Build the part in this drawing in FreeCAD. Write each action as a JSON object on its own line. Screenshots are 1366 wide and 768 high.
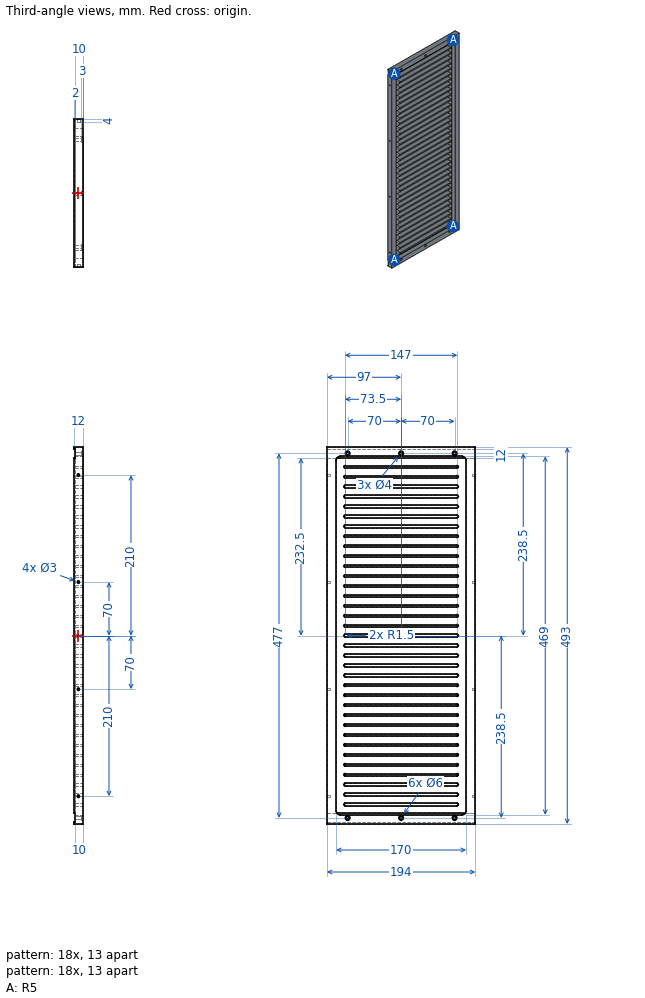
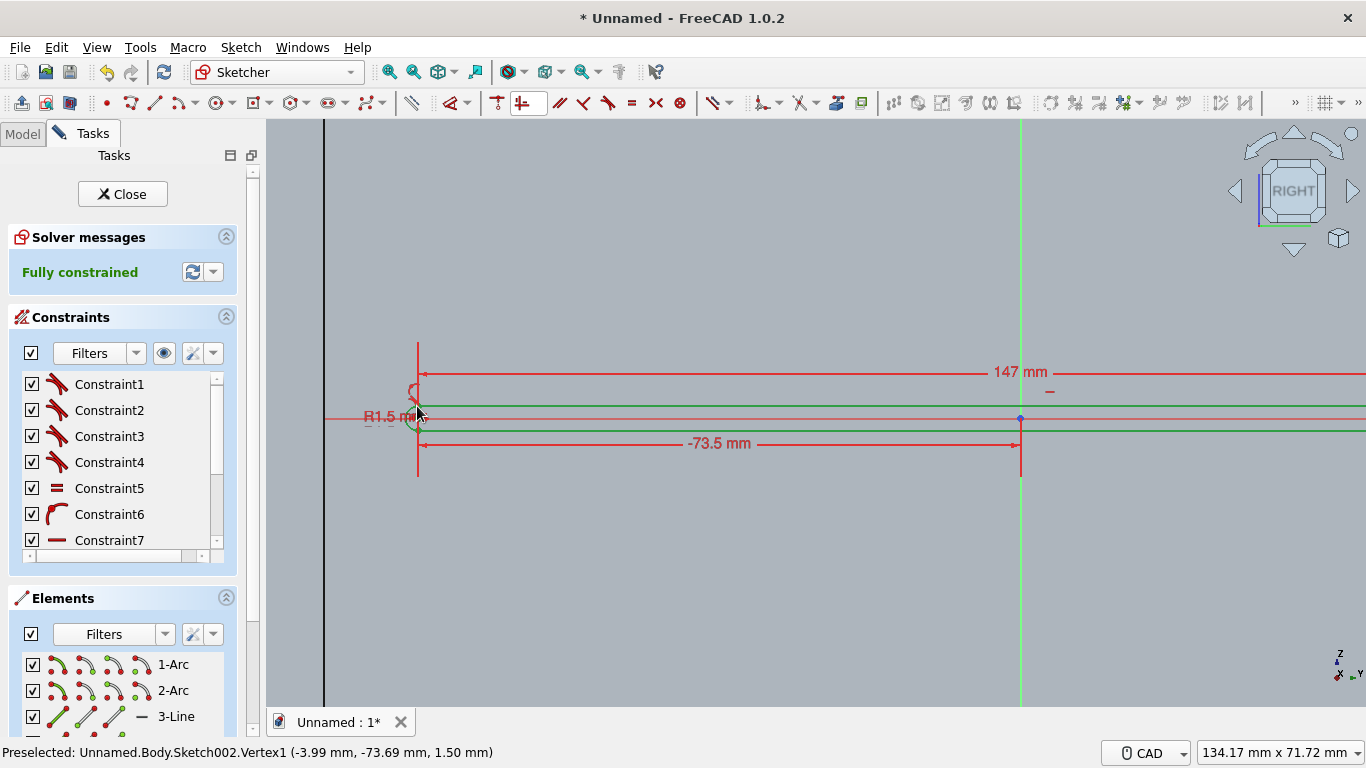
{"action": "left_click", "coordinate": [123, 194]}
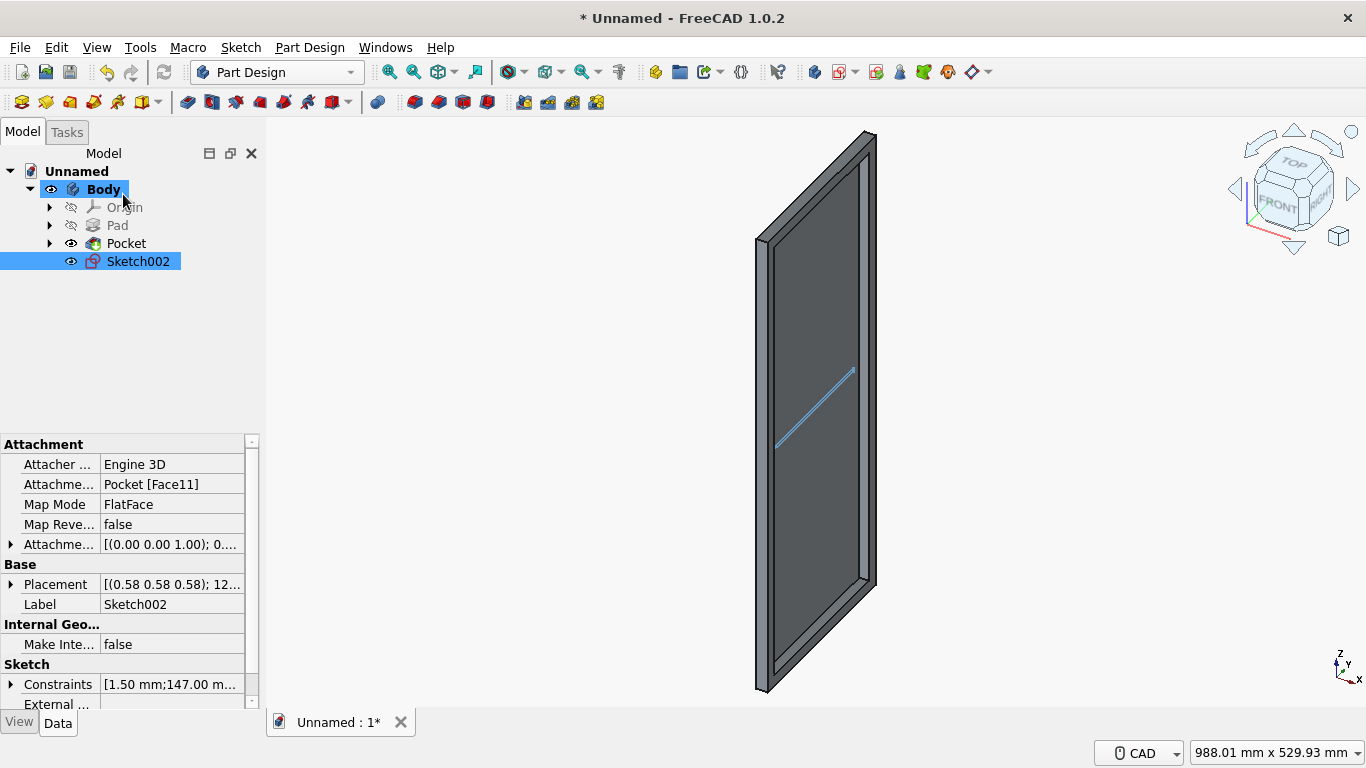
{"action": "left_click", "coordinate": [22, 102]}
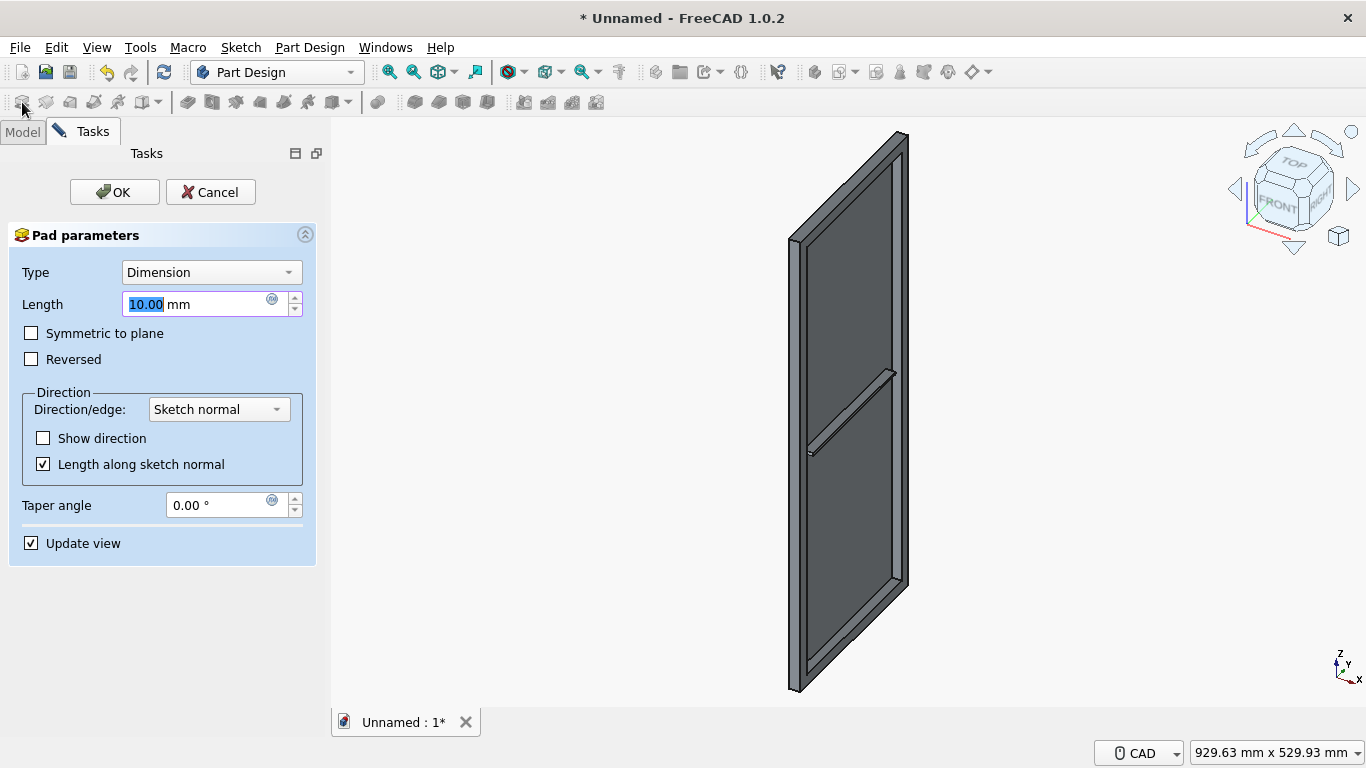
{"action": "type", "text": "10"}
{"action": "key", "text": "Tab"}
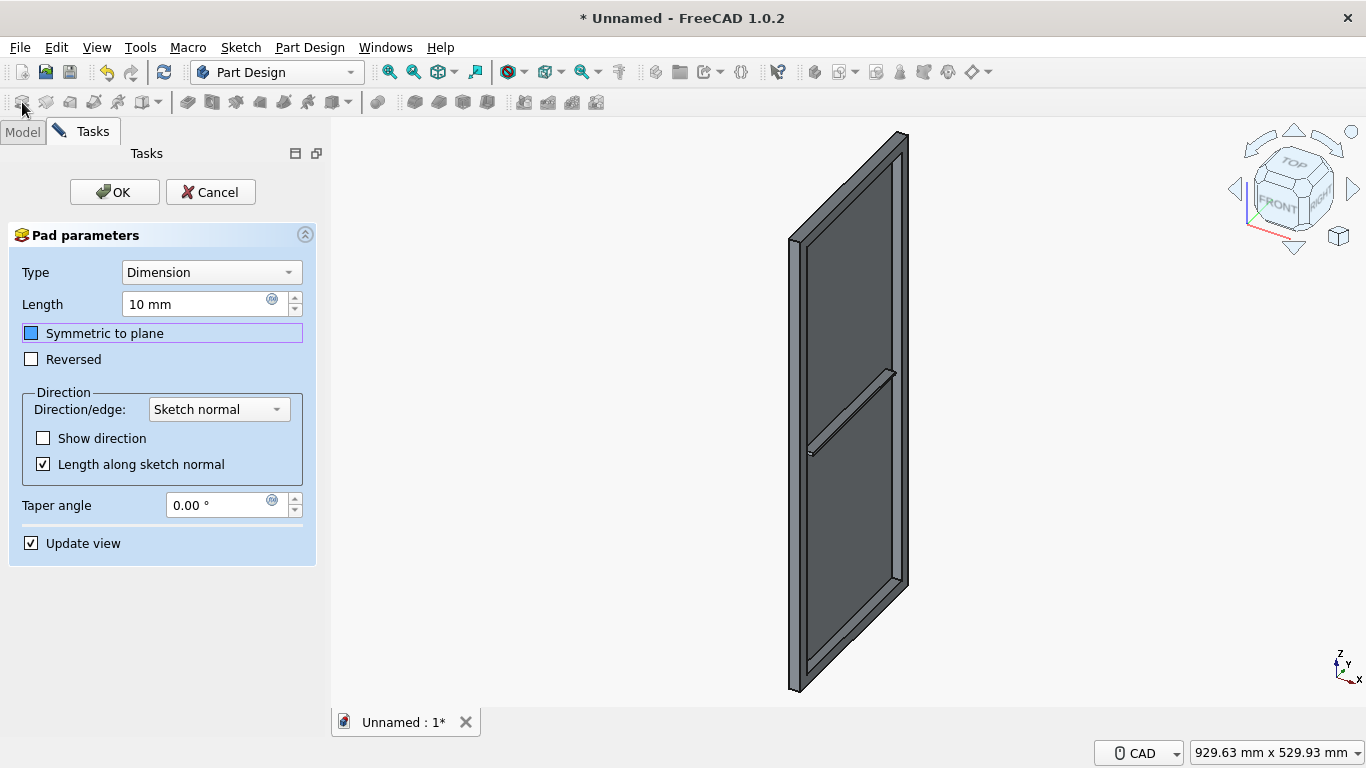
{"action": "left_click", "coordinate": [115, 192]}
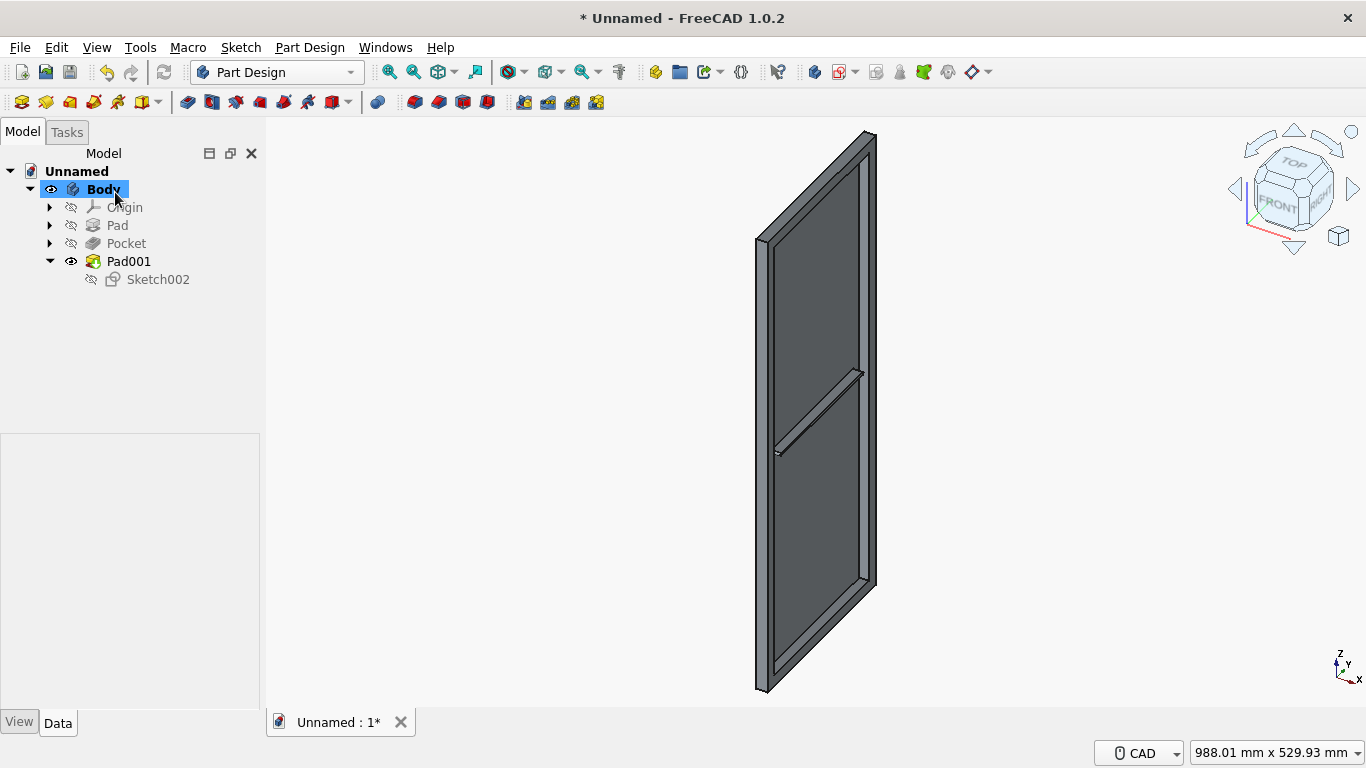
{"action": "left_click", "coordinate": [116, 261]}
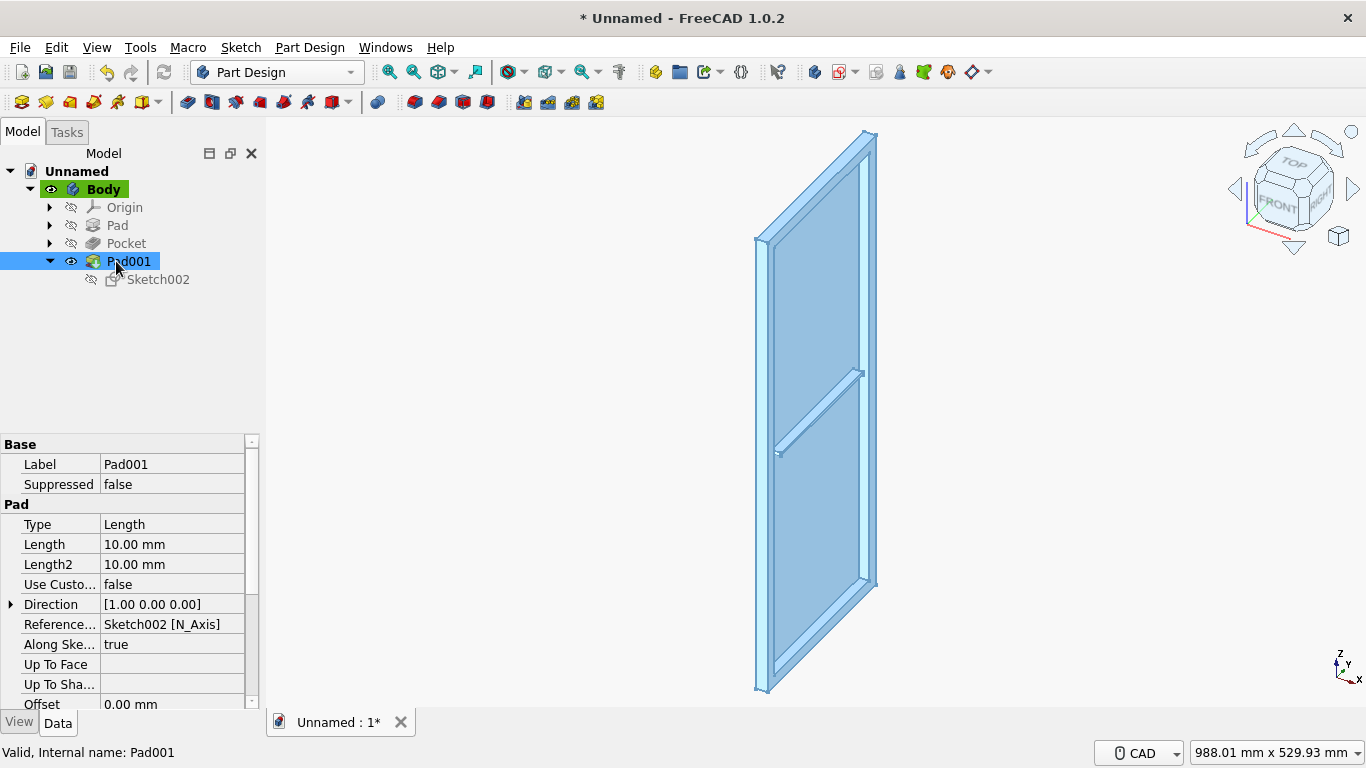
{"action": "left_click", "coordinate": [548, 102]}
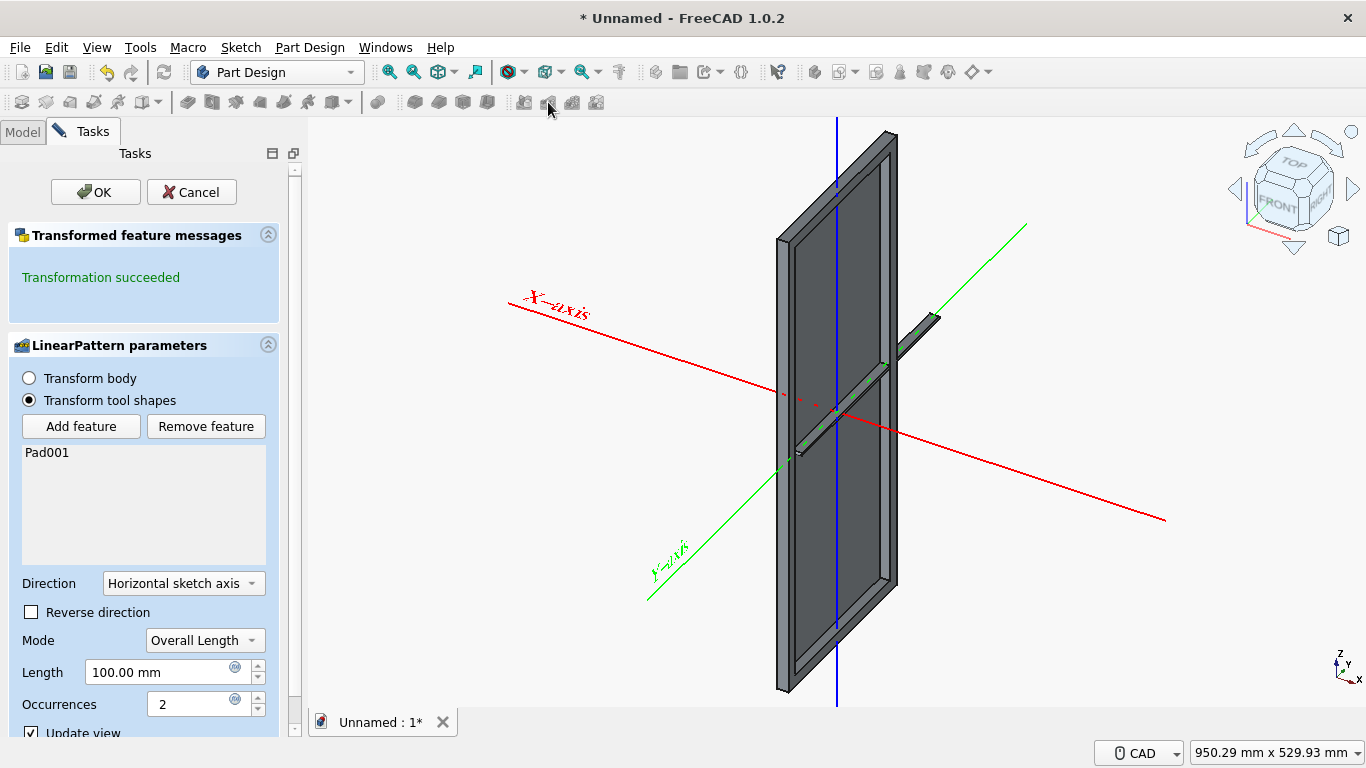
{"action": "left_click", "coordinate": [184, 584]}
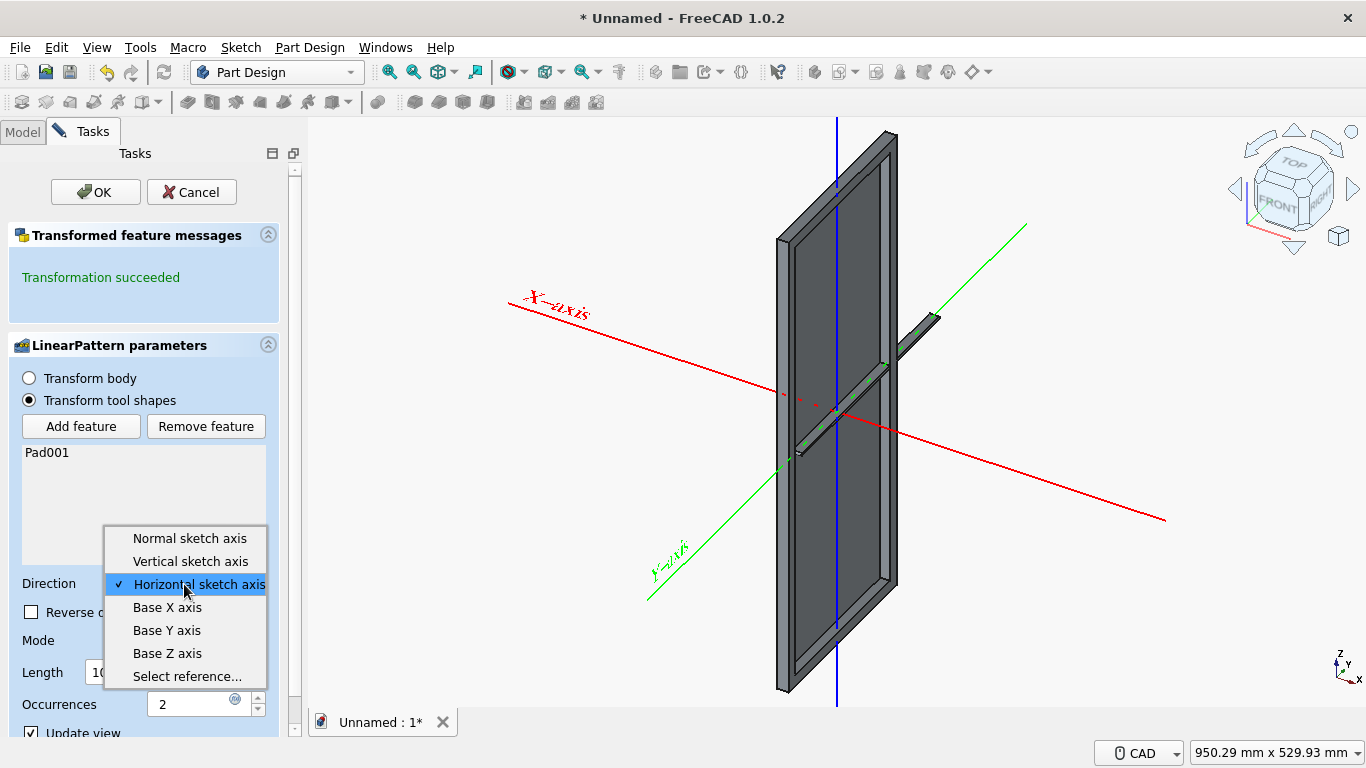
{"action": "left_click", "coordinate": [184, 654]}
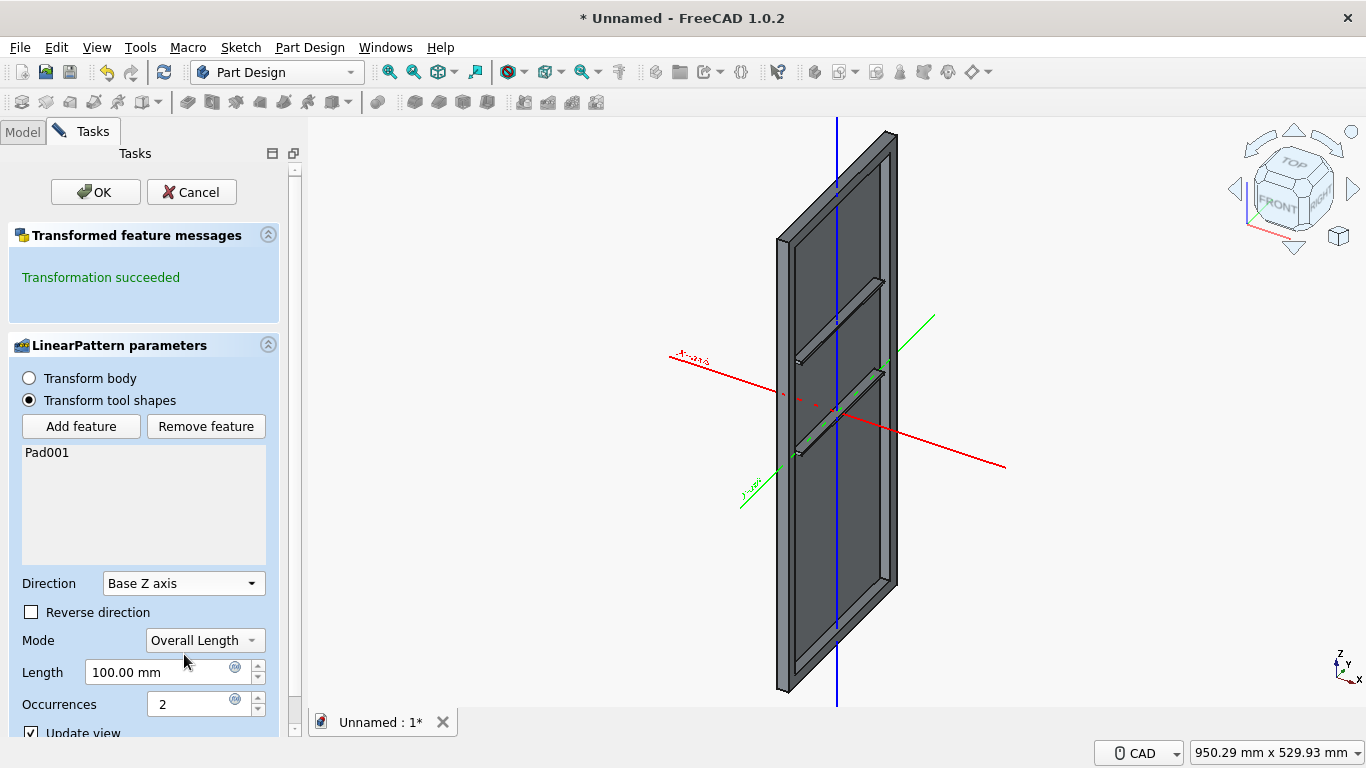
{"action": "left_click", "coordinate": [206, 640]}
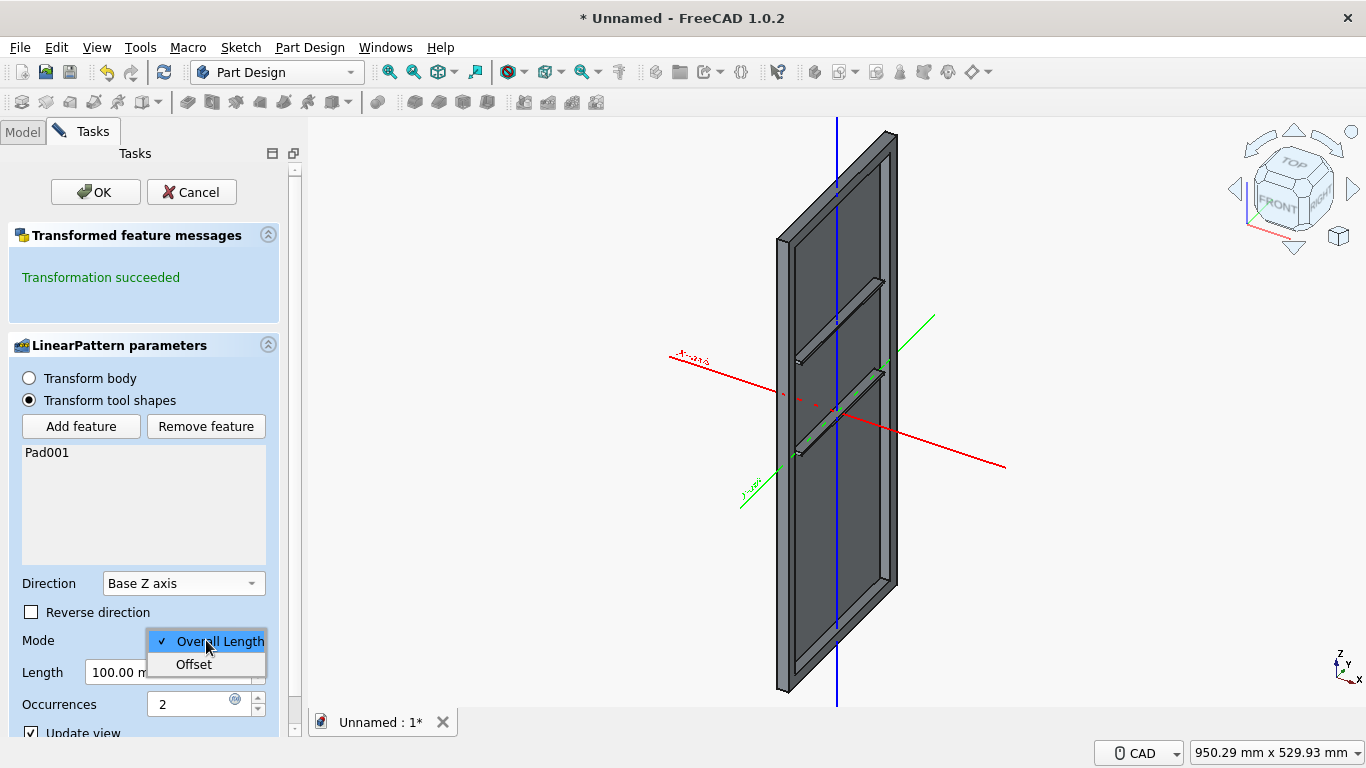
{"action": "left_click", "coordinate": [206, 664]}